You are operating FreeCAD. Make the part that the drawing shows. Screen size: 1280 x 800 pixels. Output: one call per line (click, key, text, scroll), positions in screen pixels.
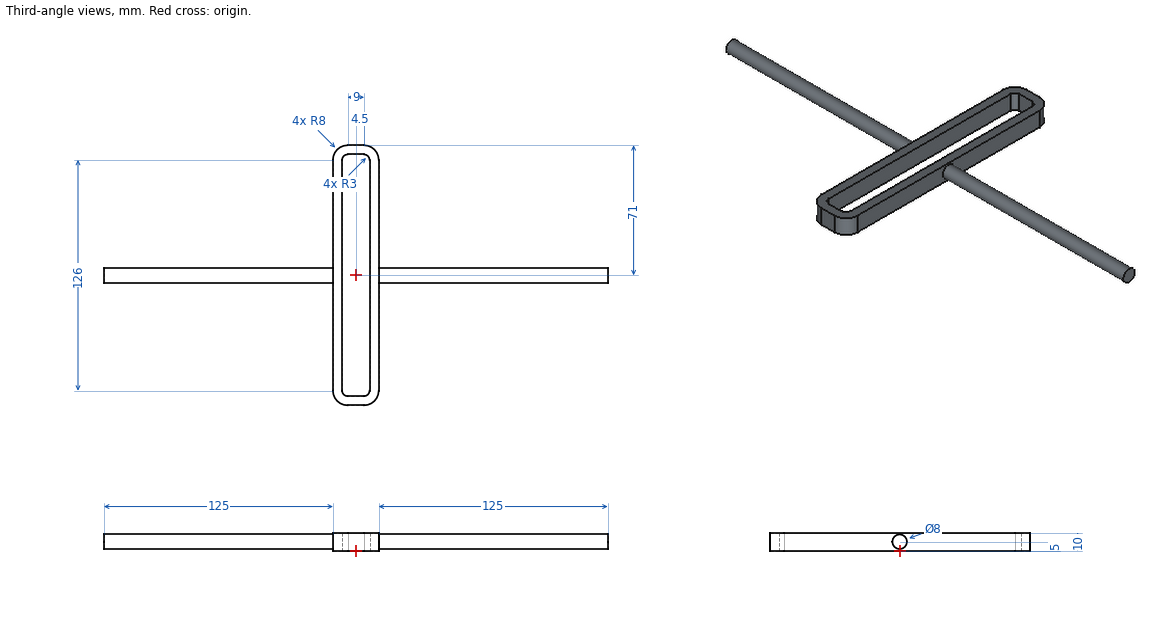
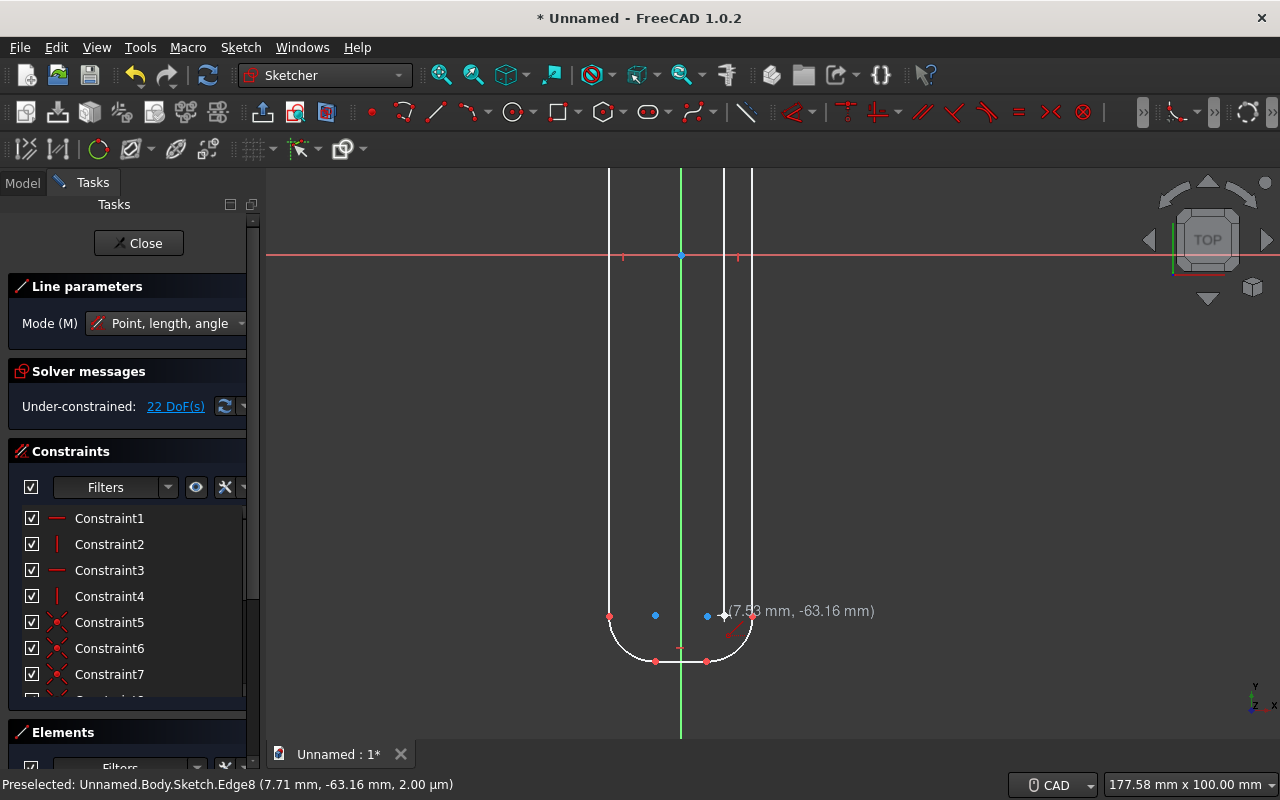
click(707, 632)
click(655, 632)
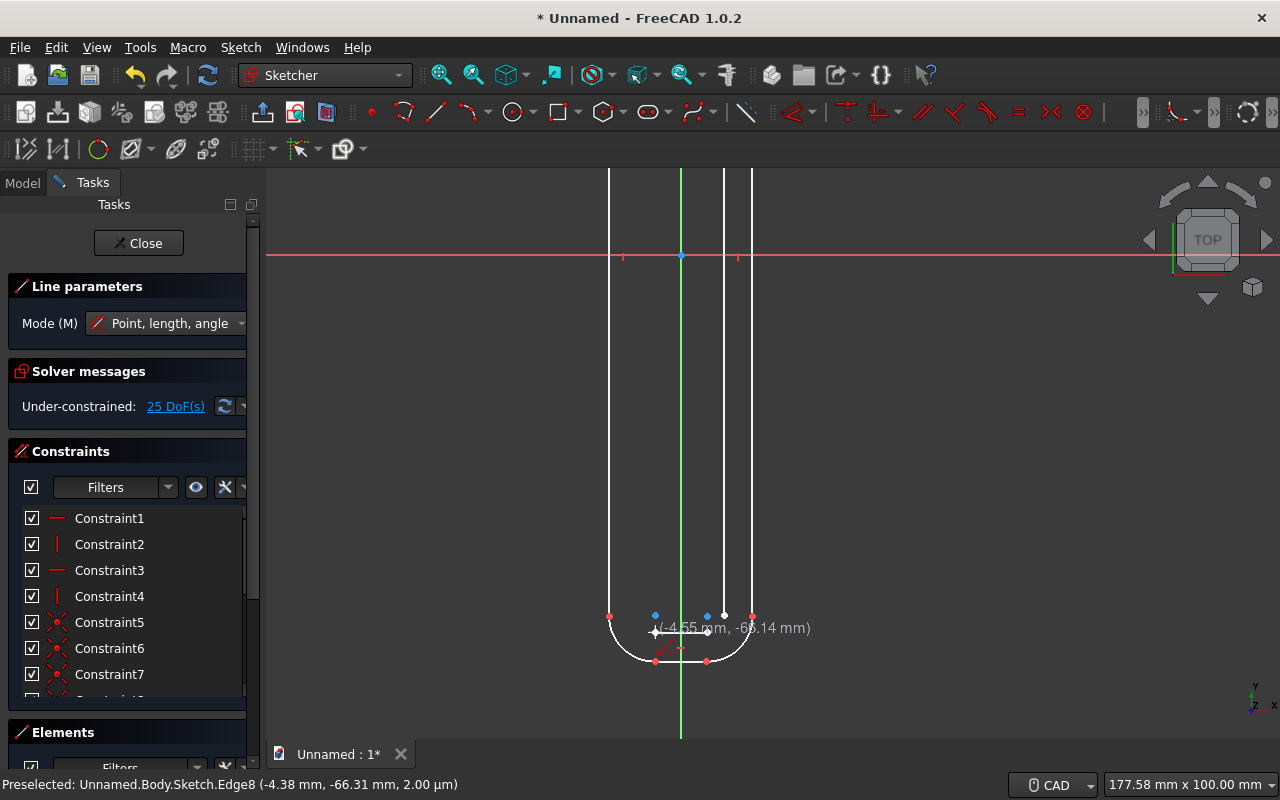
click(638, 615)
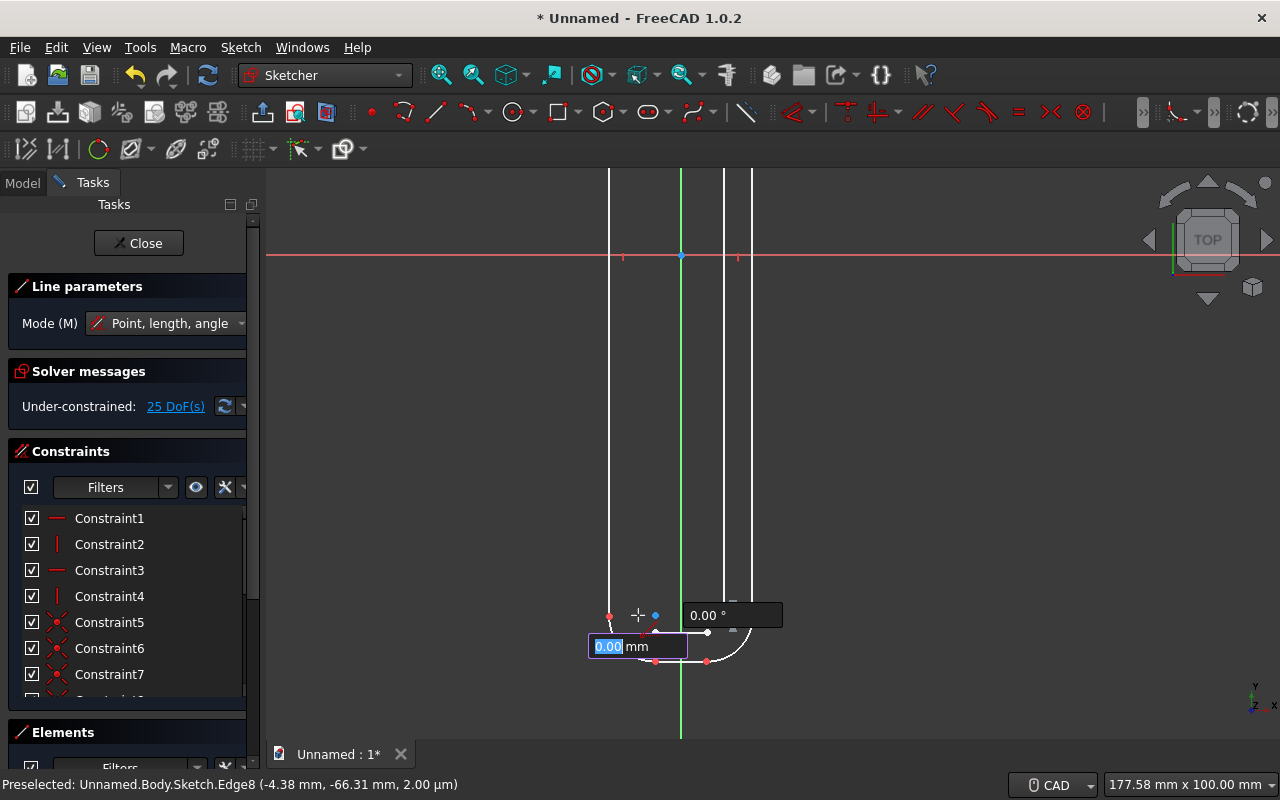
scroll(724, 615, down, 4)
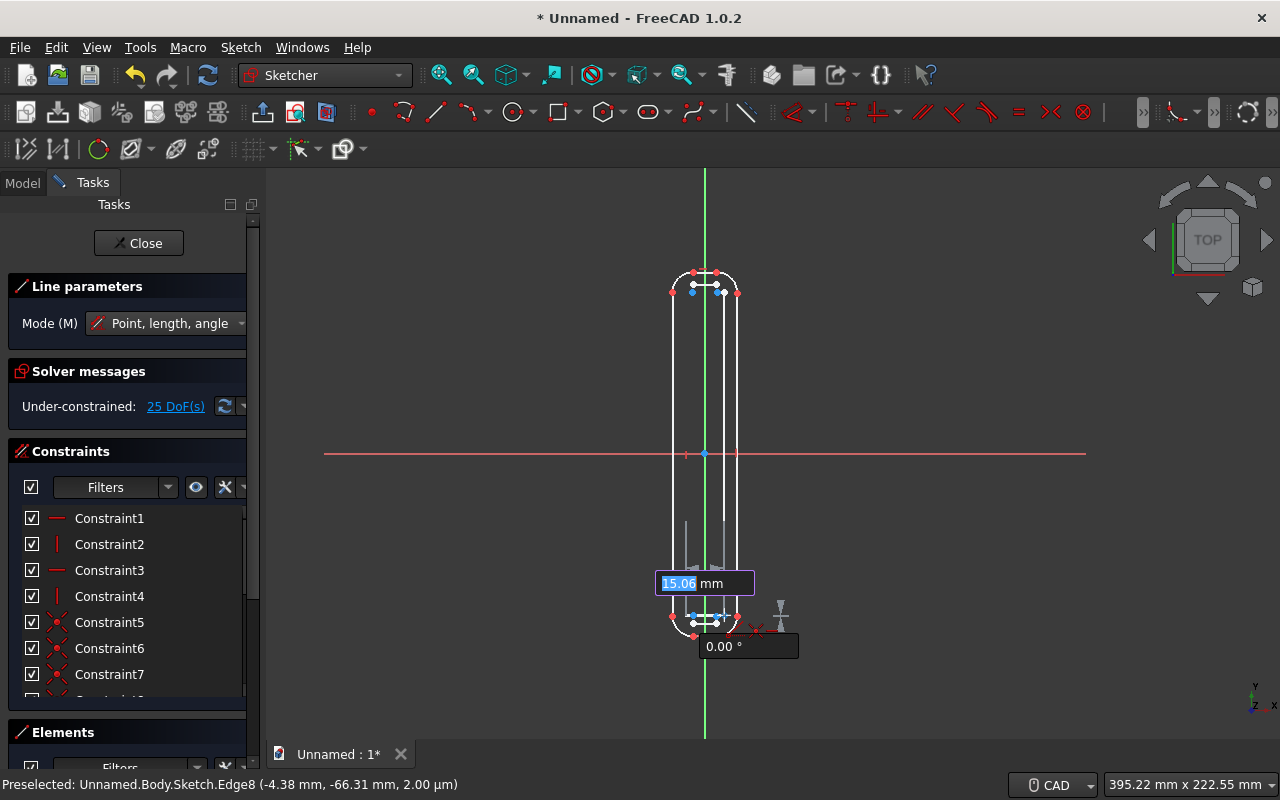
scroll(686, 292, up, 4)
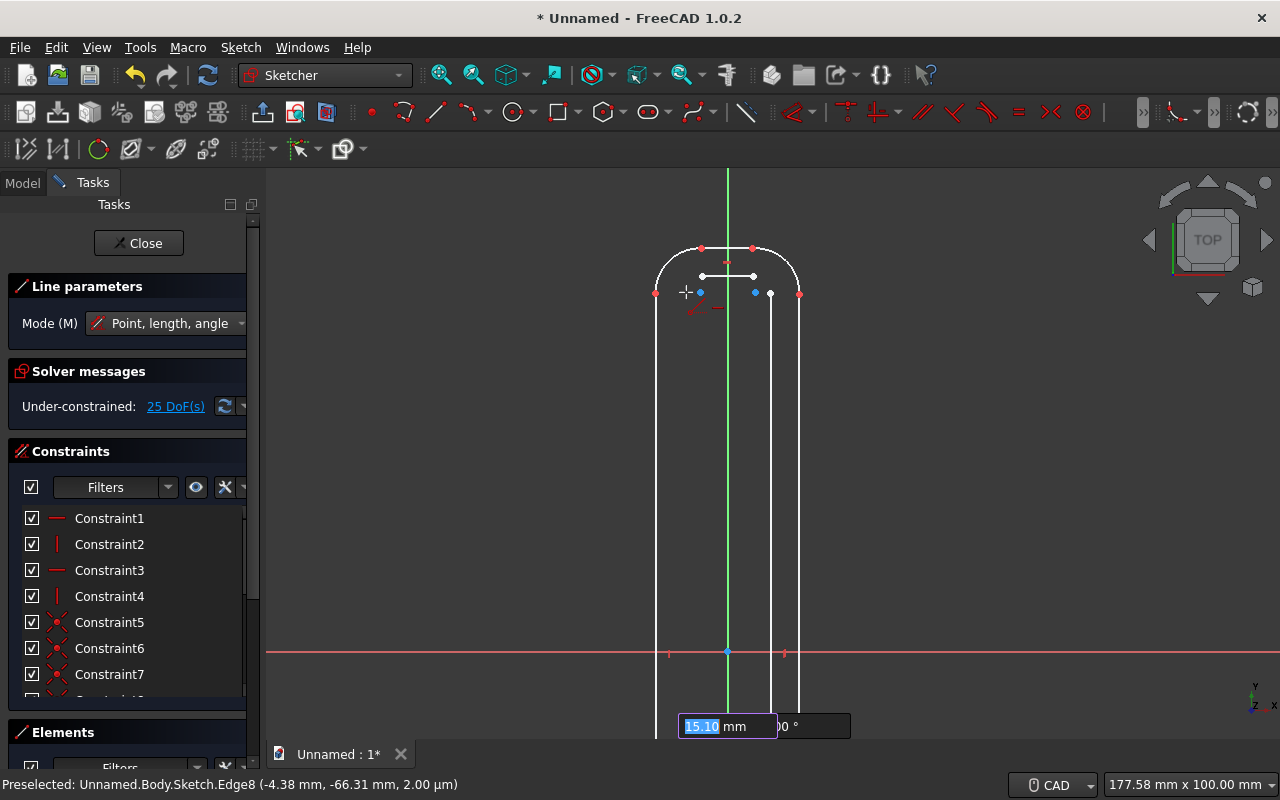
click(685, 292)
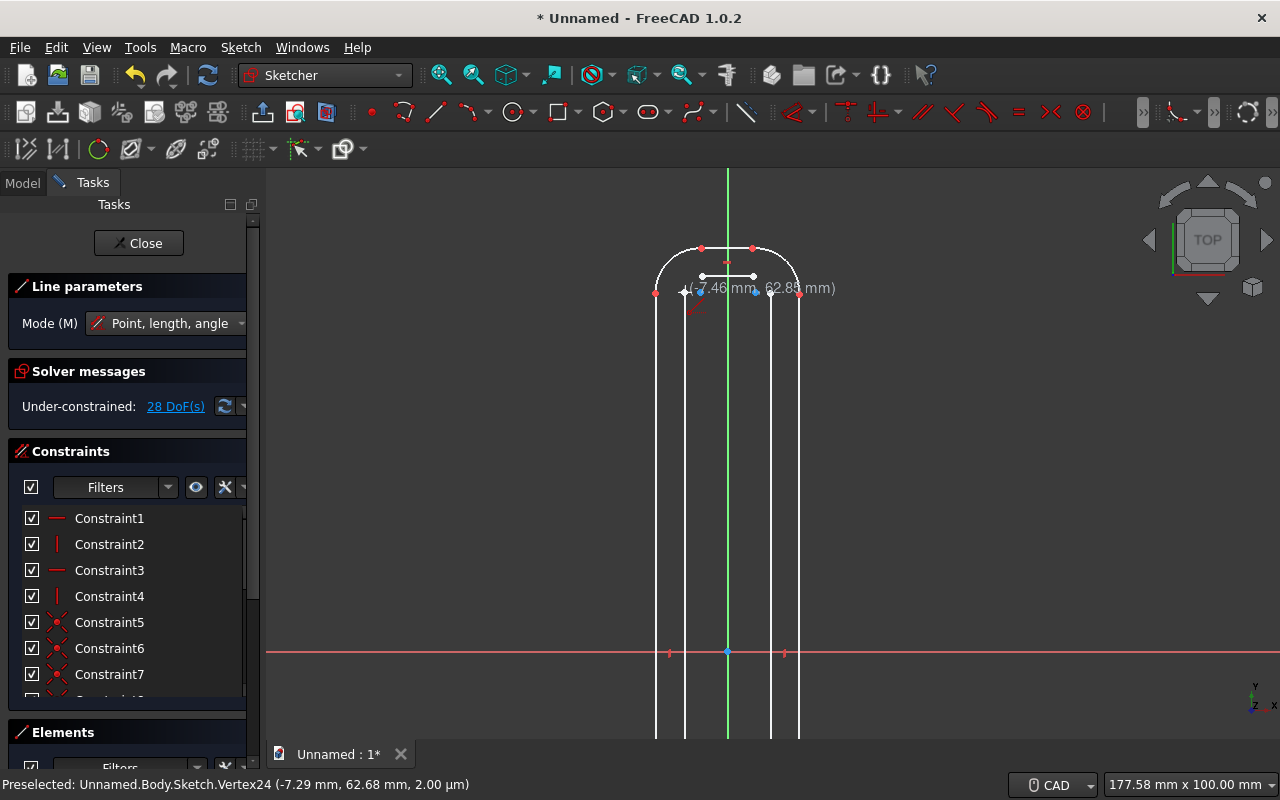
click(468, 112)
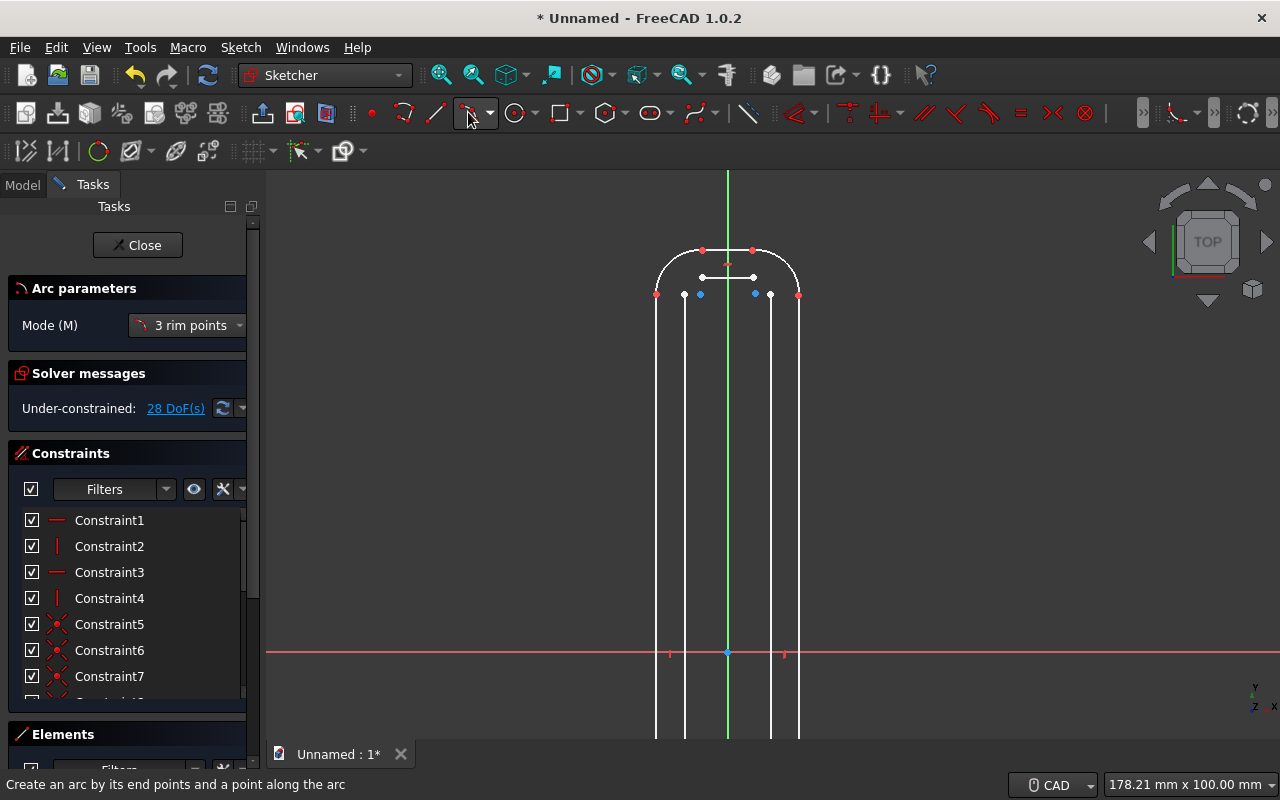
click(754, 278)
click(771, 295)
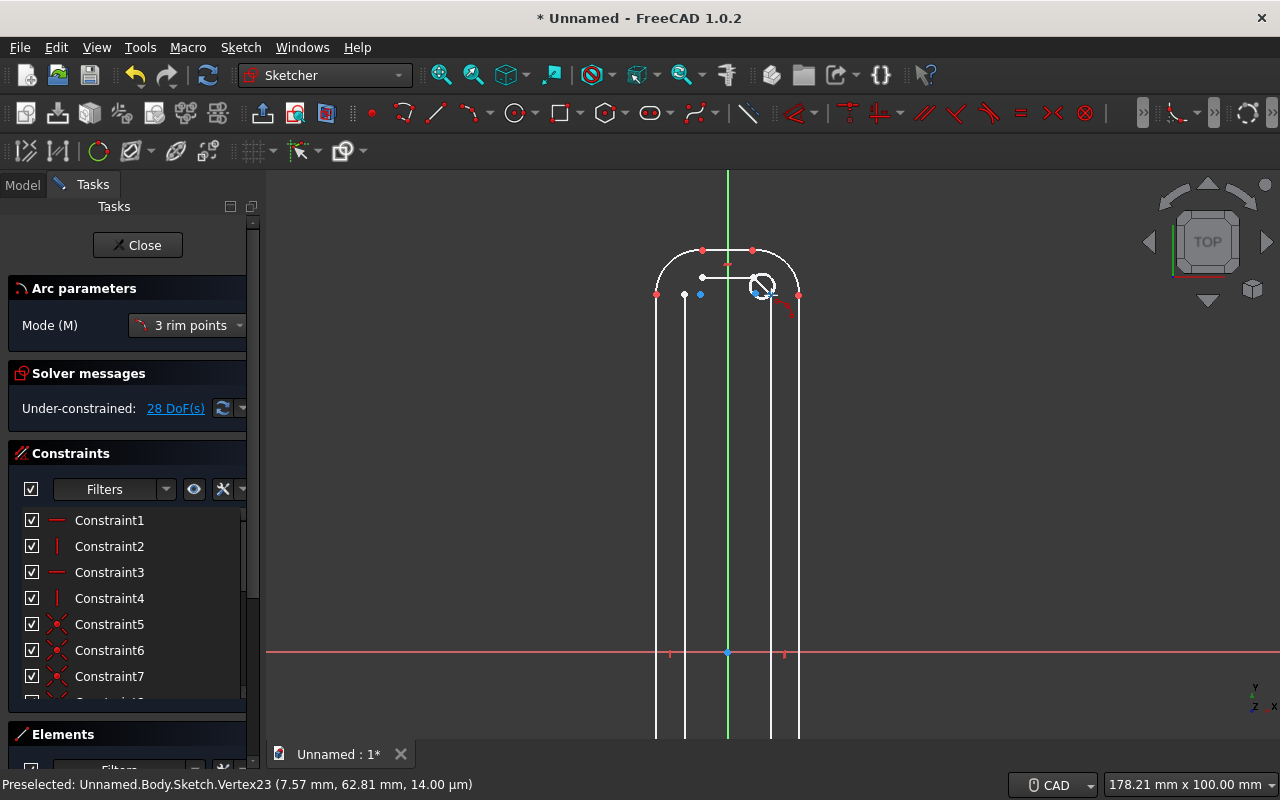
scroll(765, 282, up, 6)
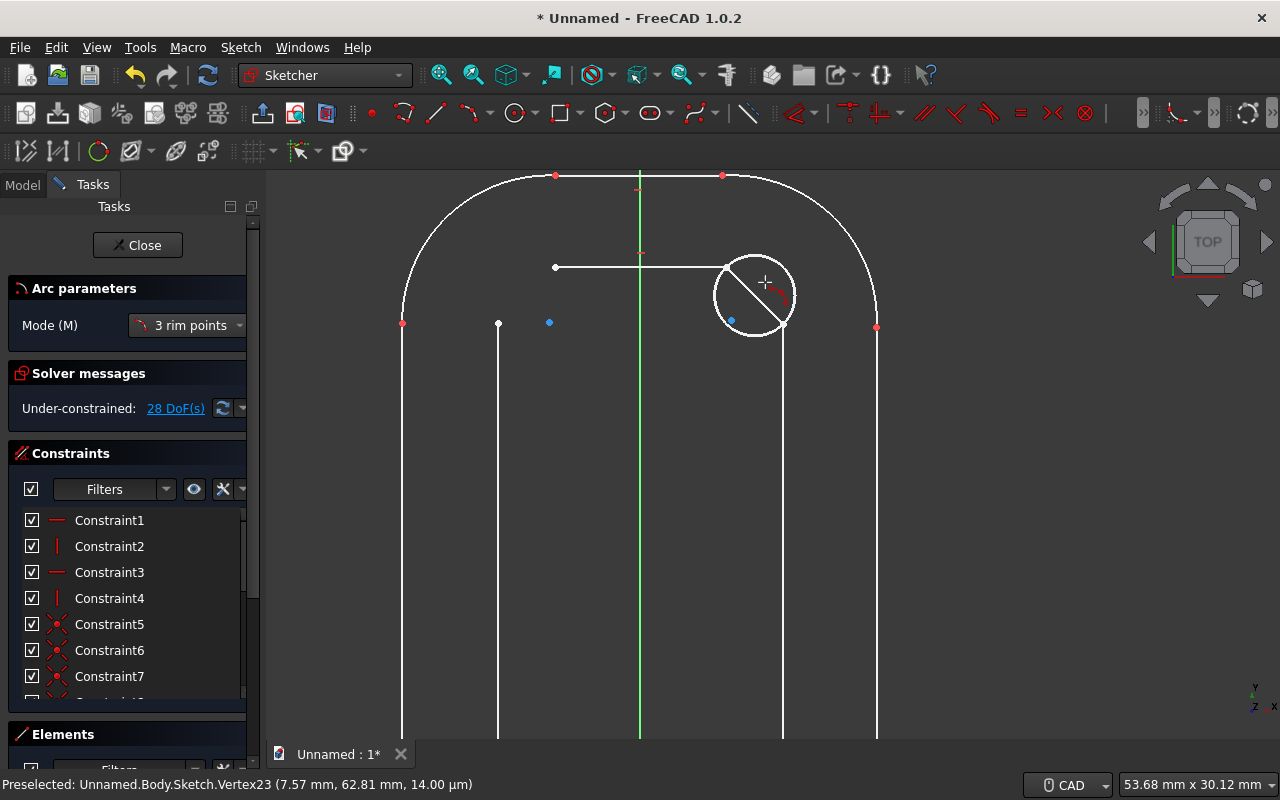
click(765, 280)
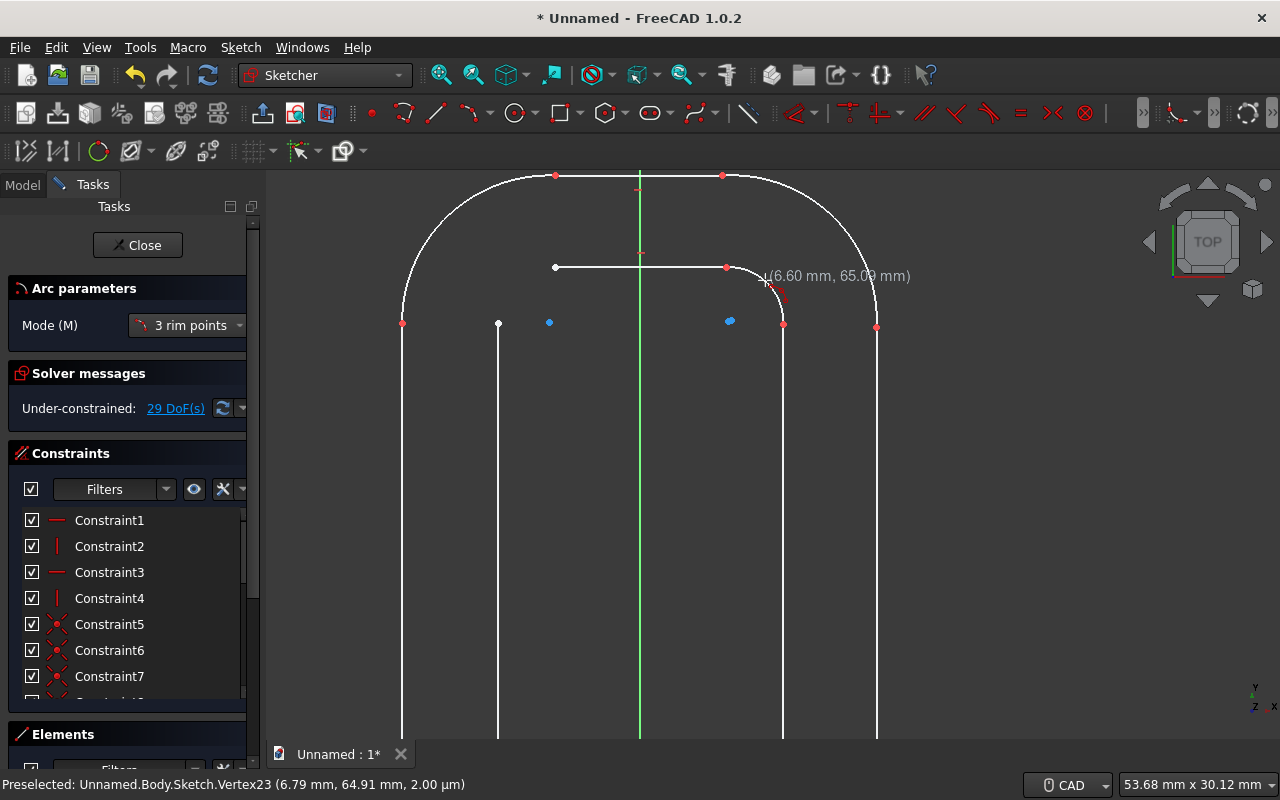
scroll(715, 289, down, 10)